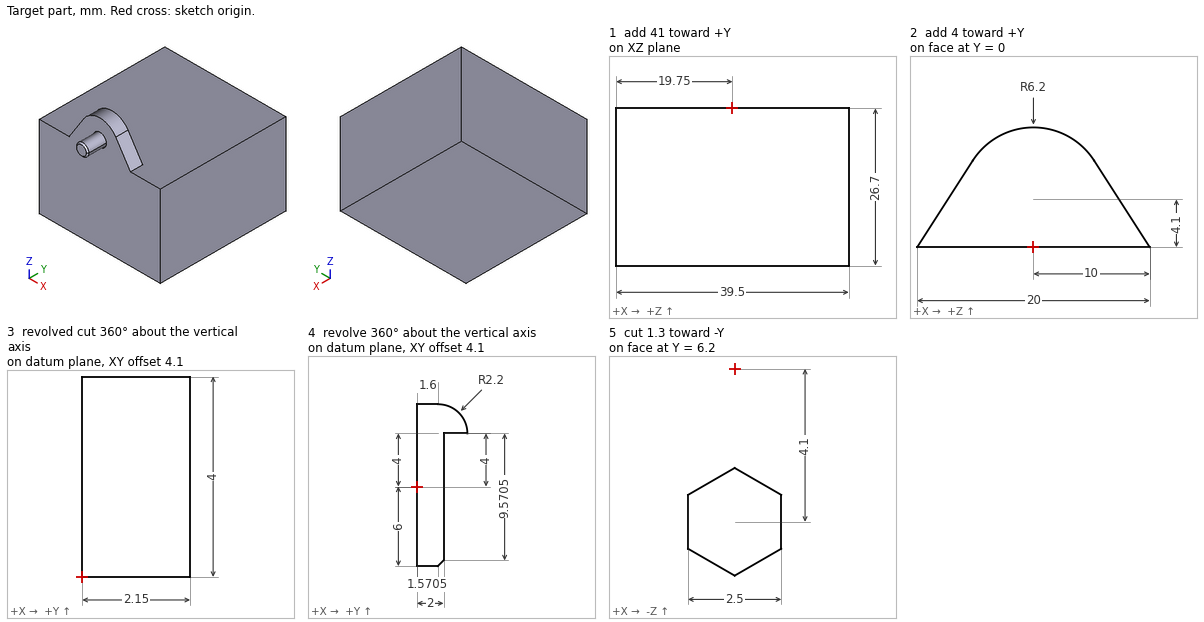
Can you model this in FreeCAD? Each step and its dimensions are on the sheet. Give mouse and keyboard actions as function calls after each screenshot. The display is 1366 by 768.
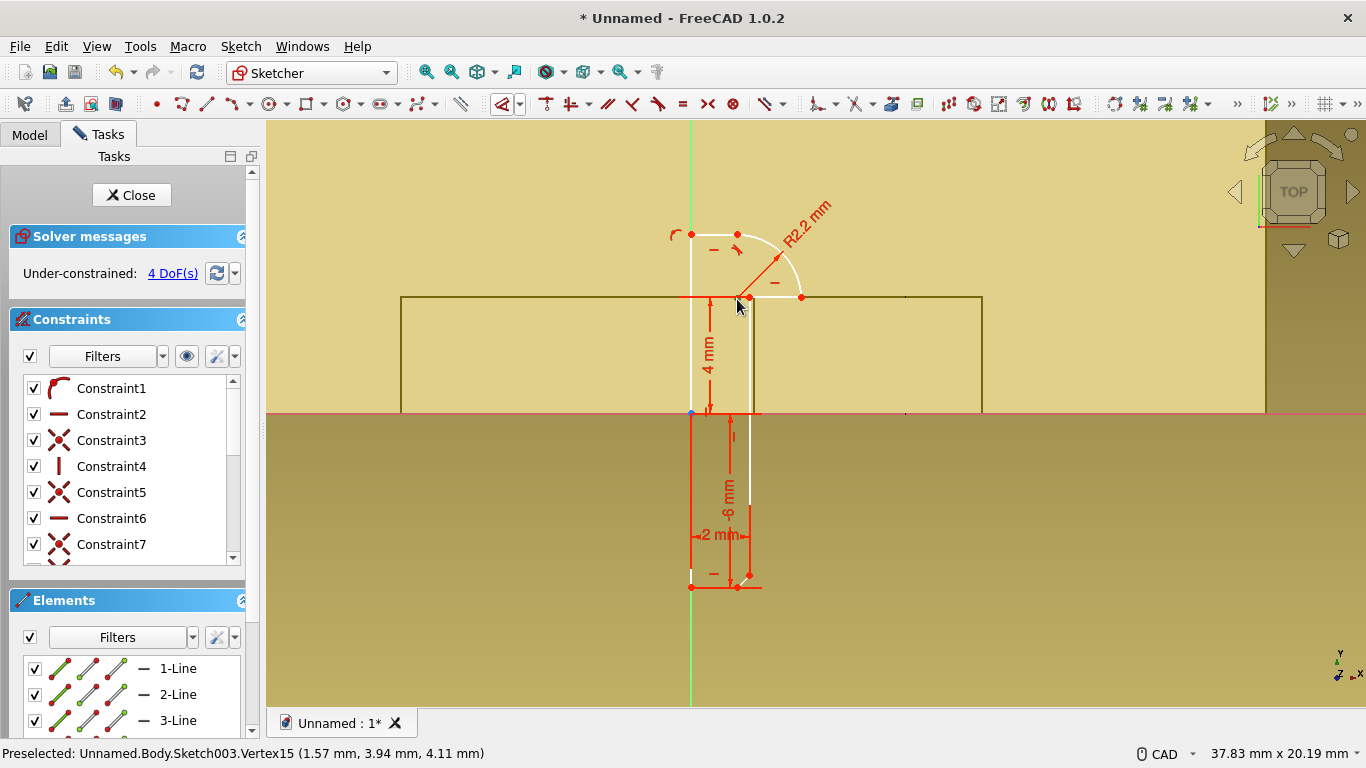
key(i)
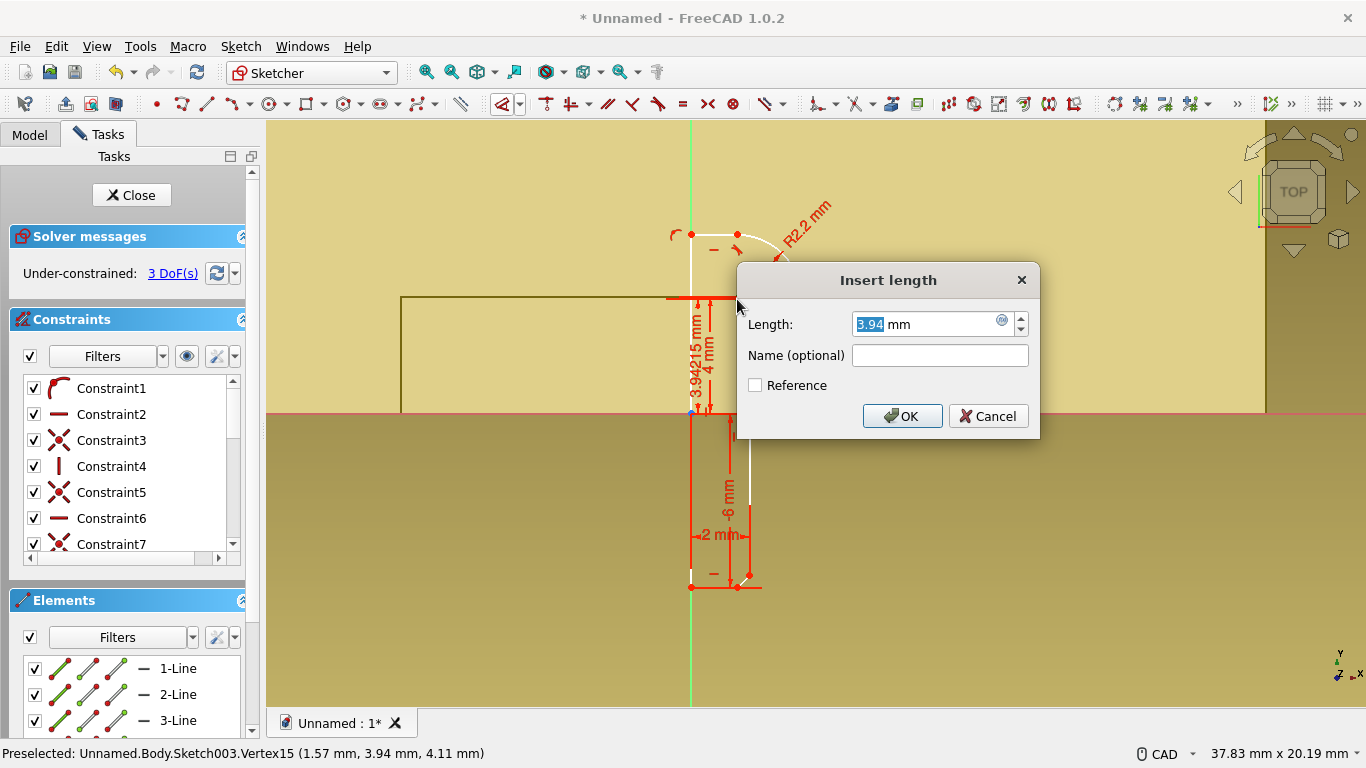
text(4)
key(Return)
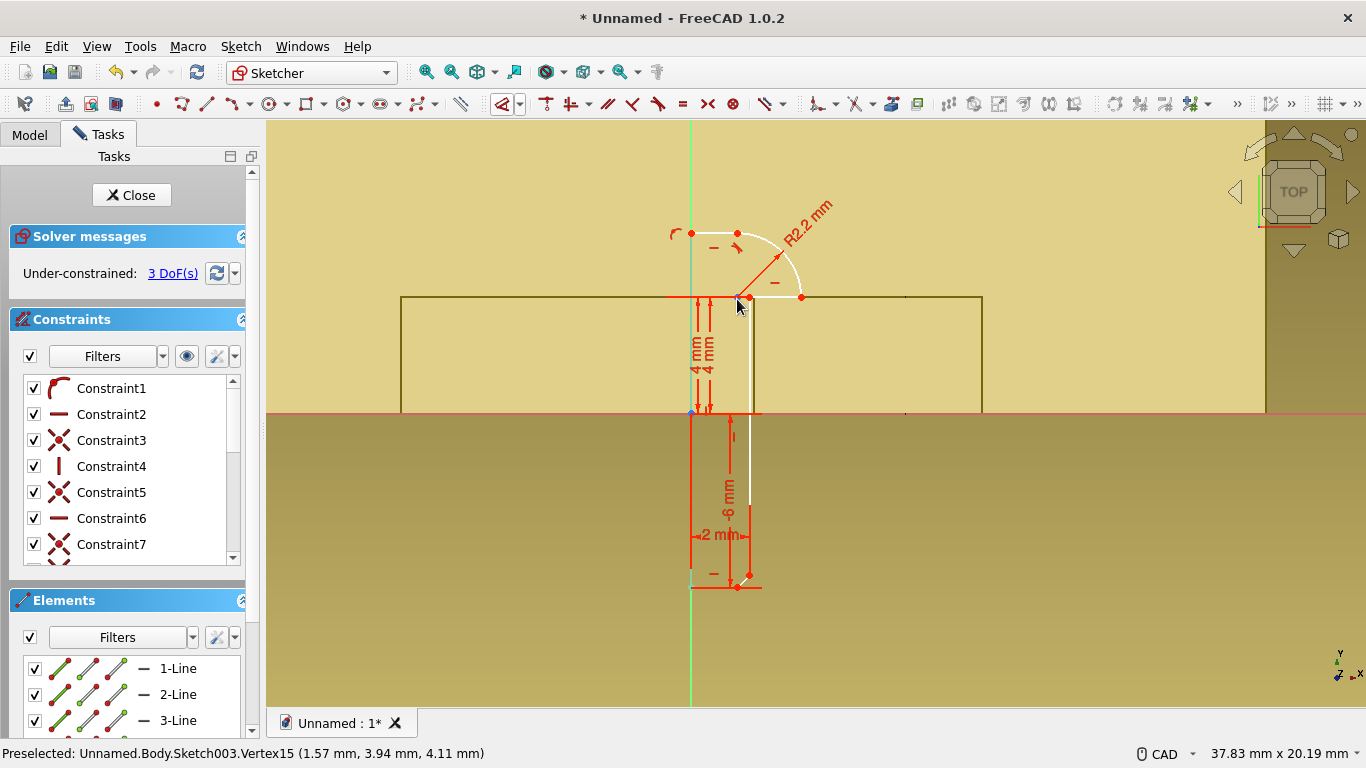
click(723, 233)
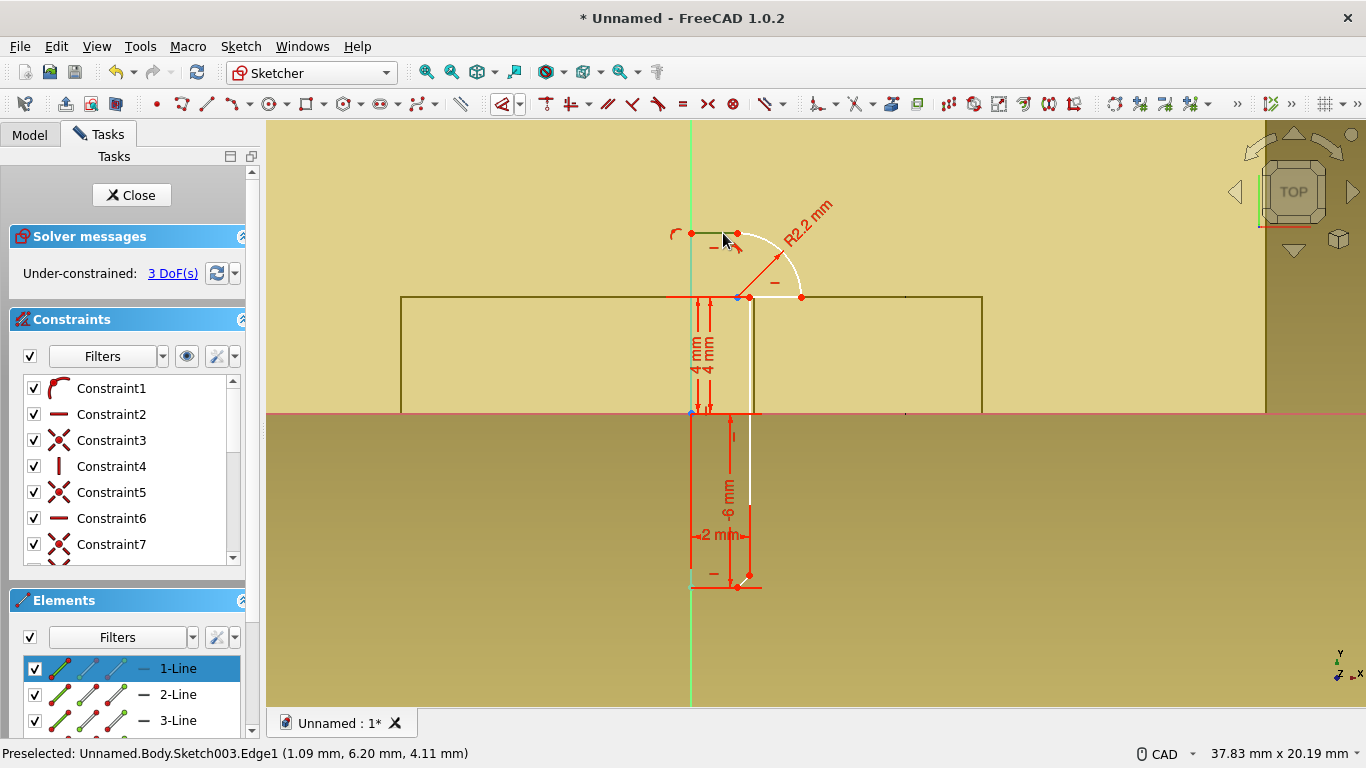
key(l)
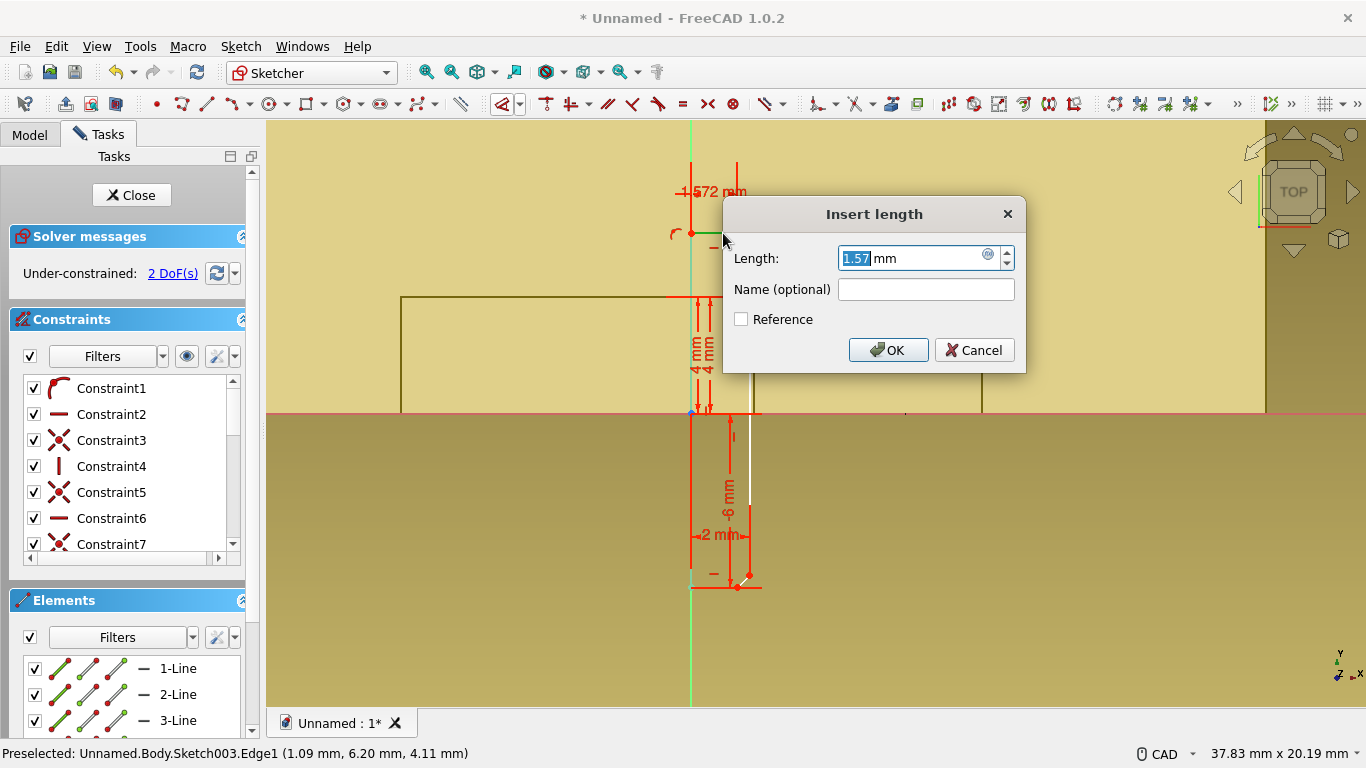
text(1.6)
key(Return)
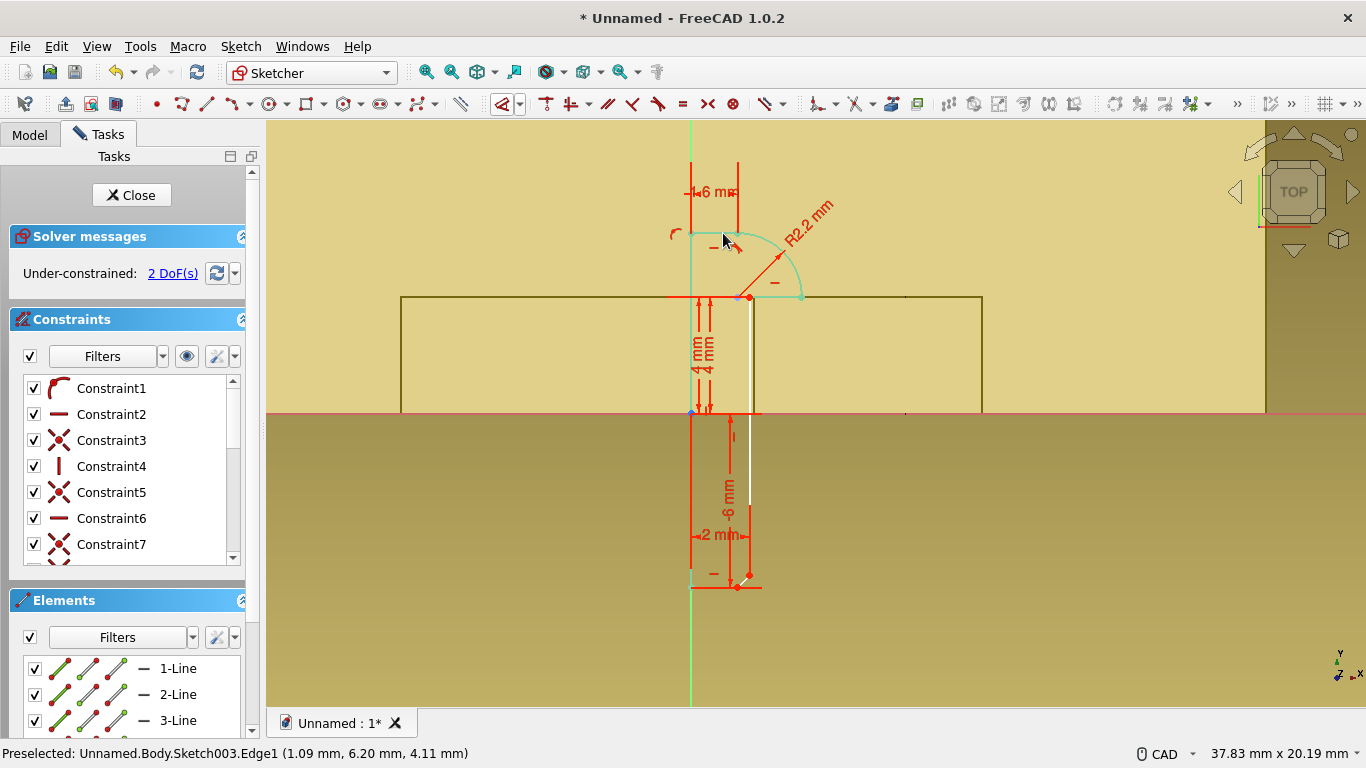
click(705, 588)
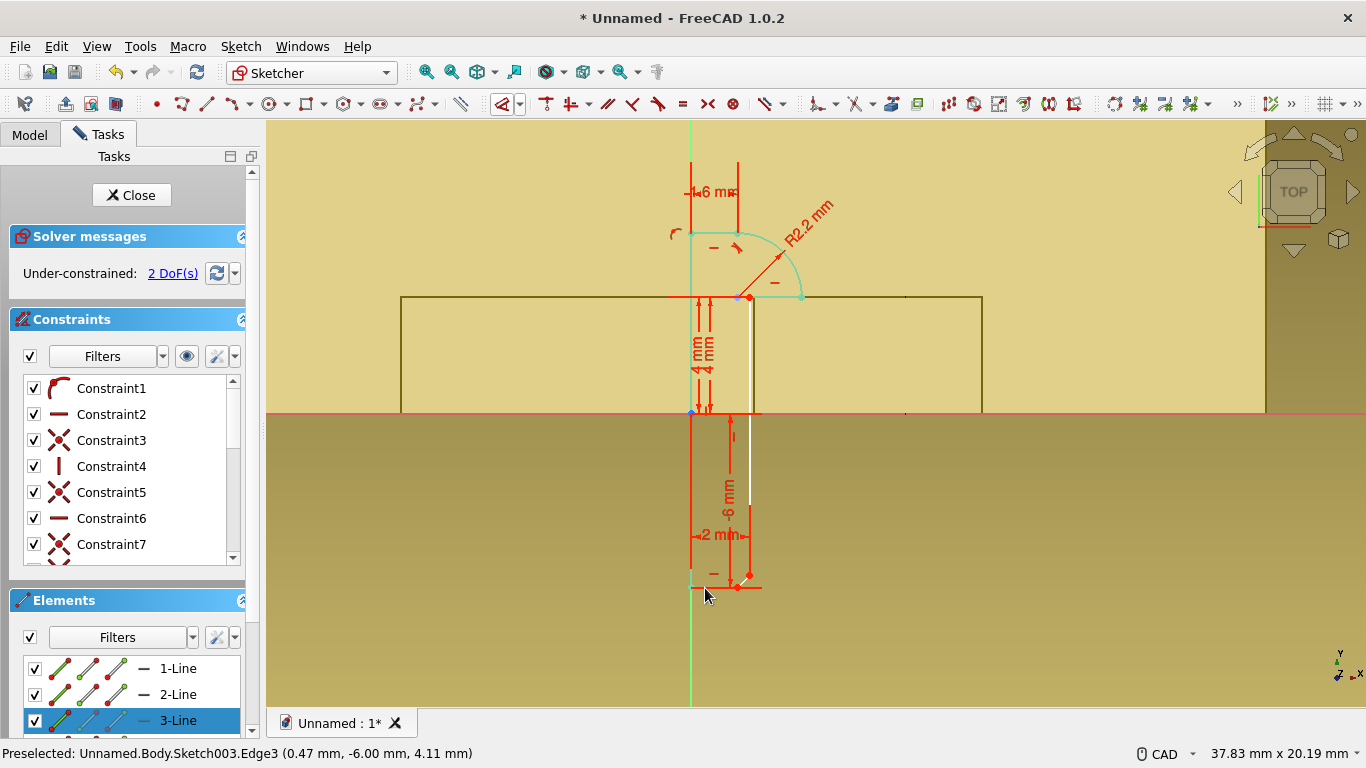
key(l)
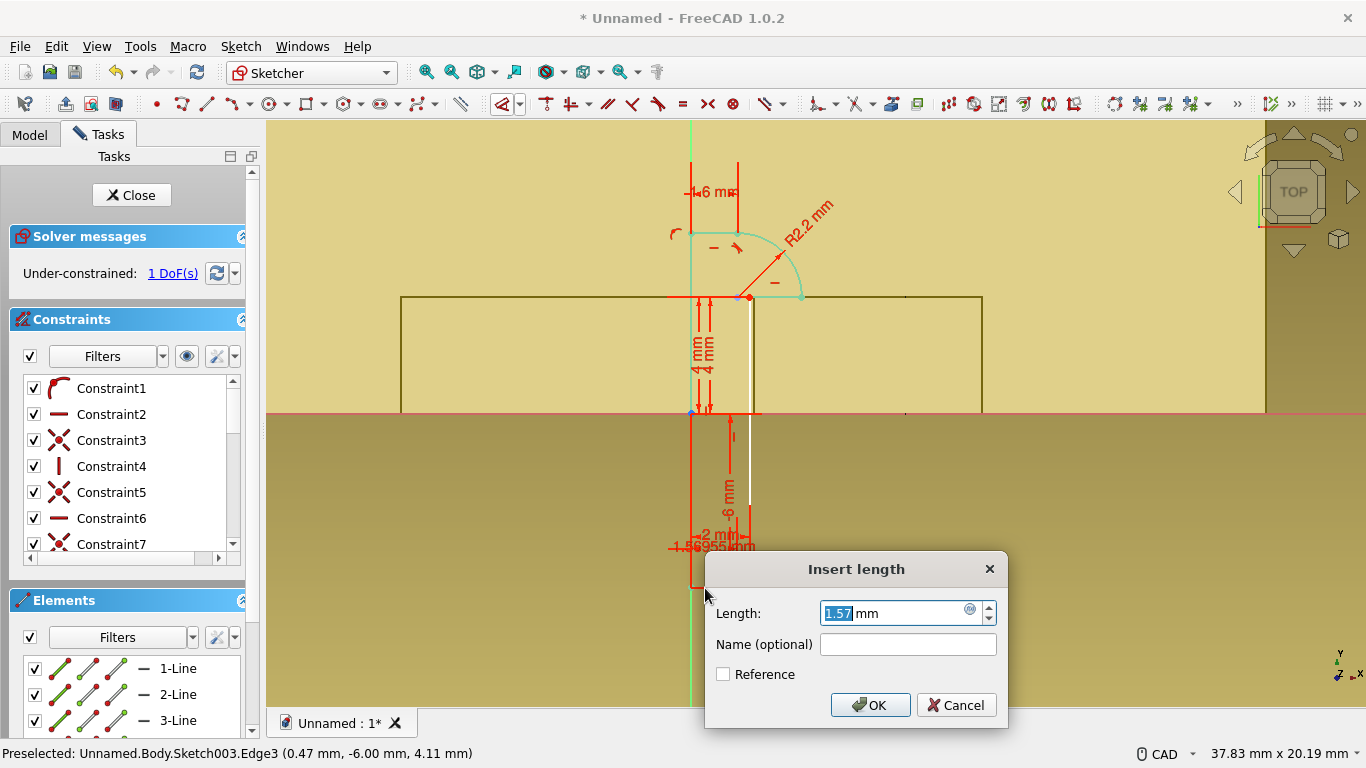
text(1.5705)
key(Return)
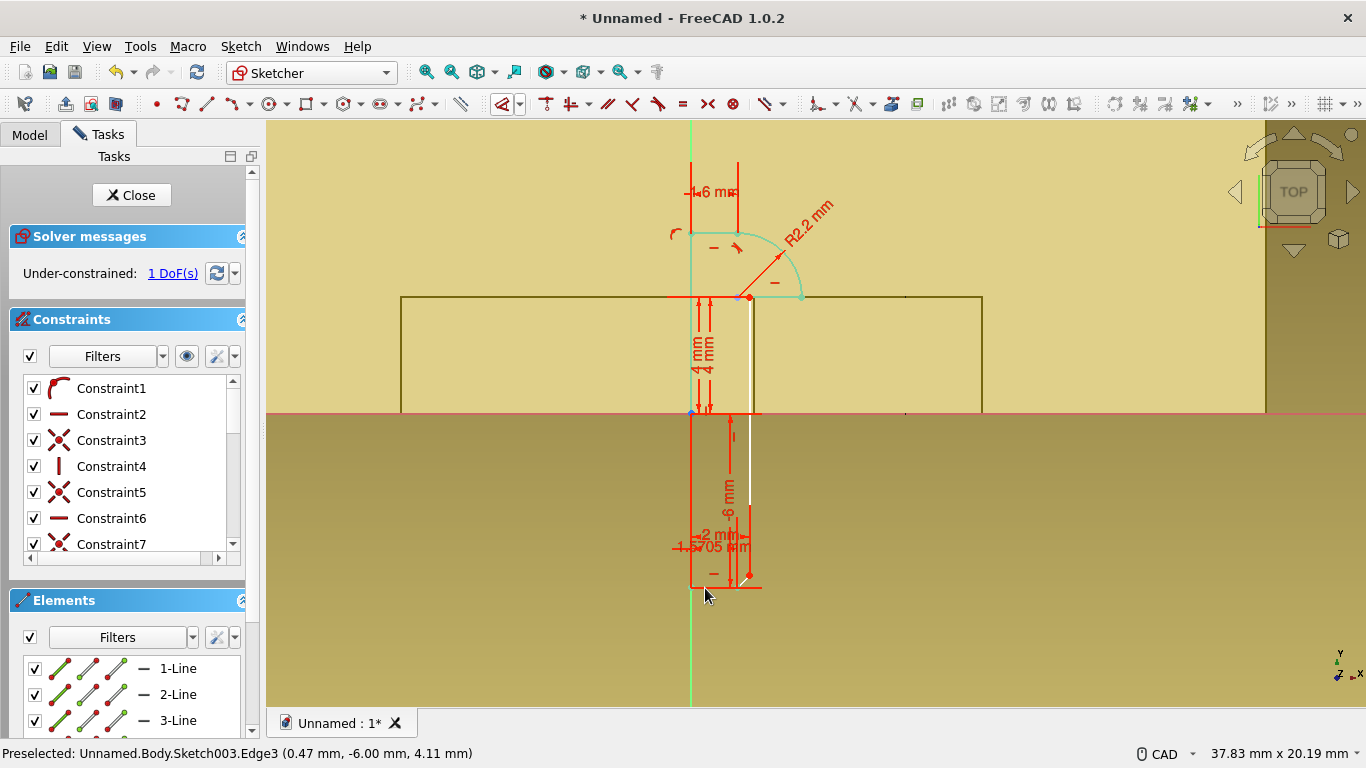
click(750, 492)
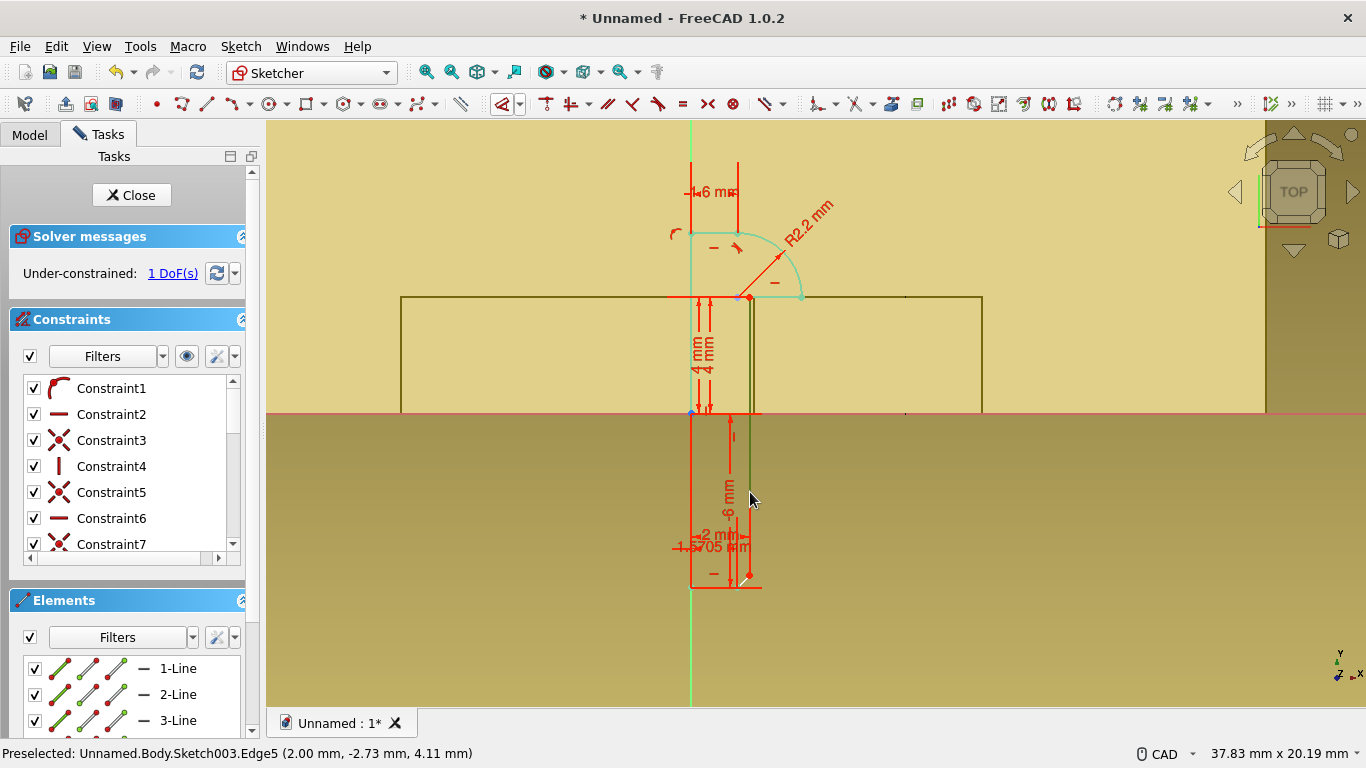
key(i)